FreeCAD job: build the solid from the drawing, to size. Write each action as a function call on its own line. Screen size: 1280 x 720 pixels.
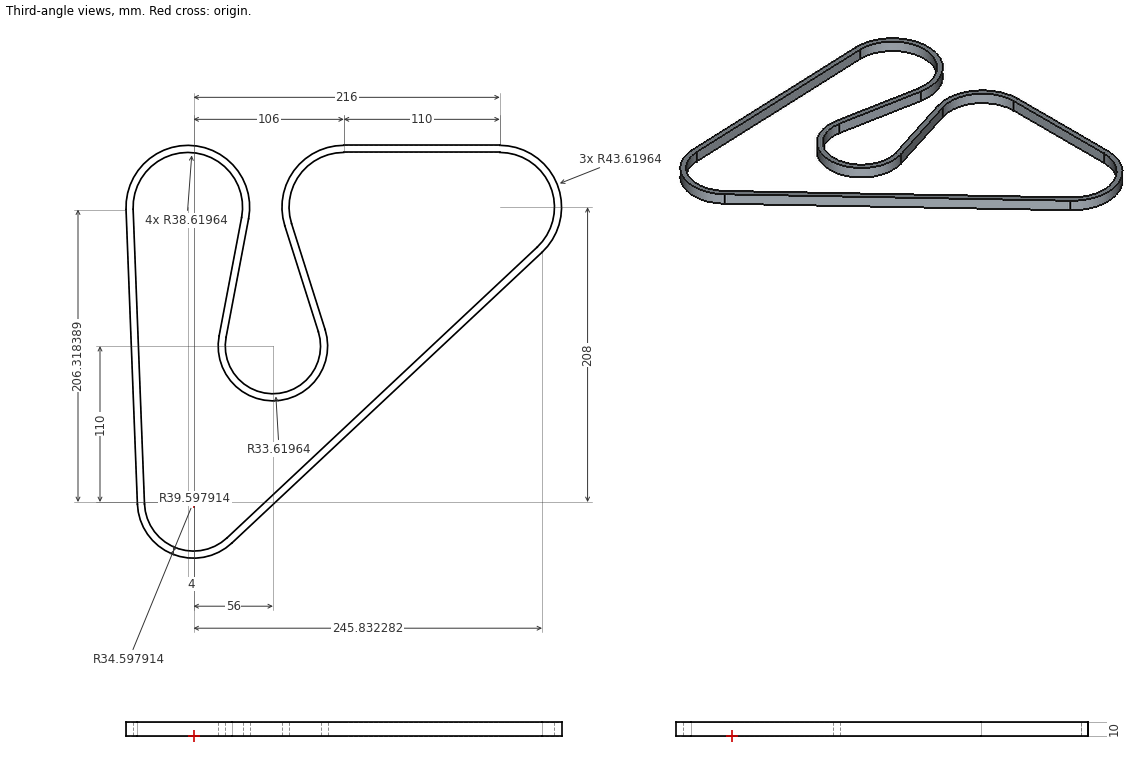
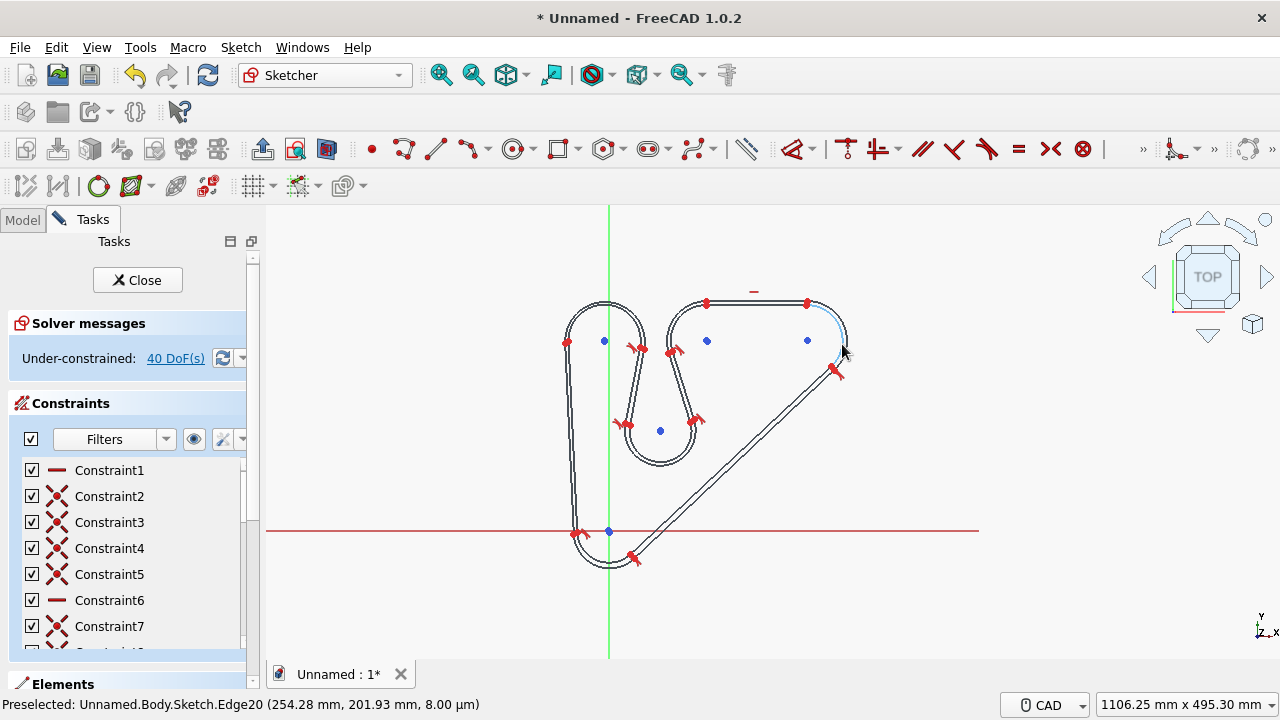
scroll(575, 475, up, 7)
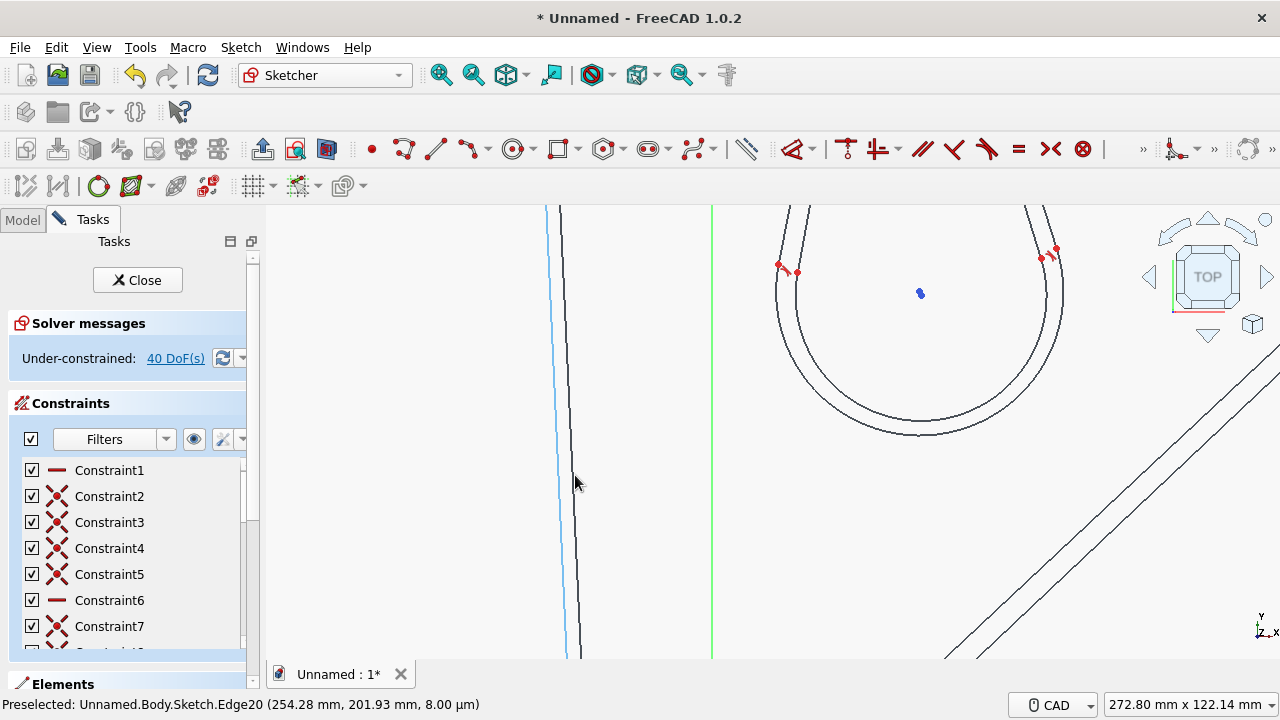
click(573, 473)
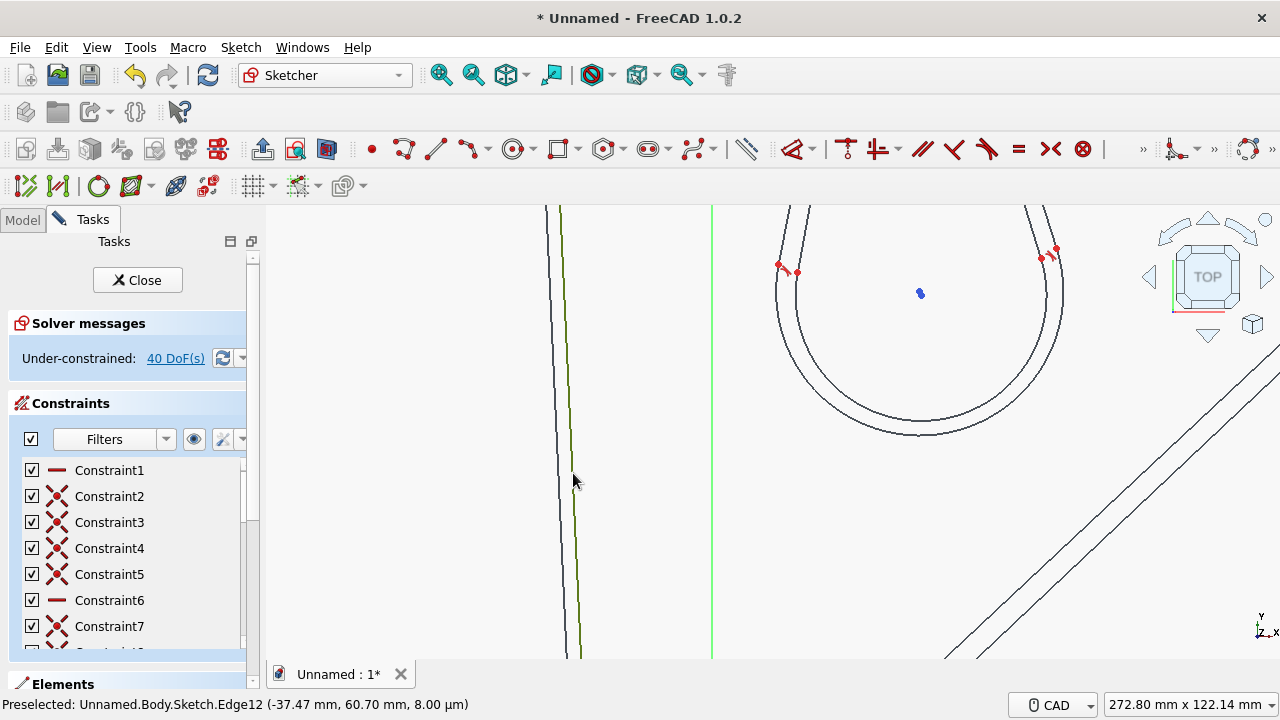
scroll(575, 475, down, 7)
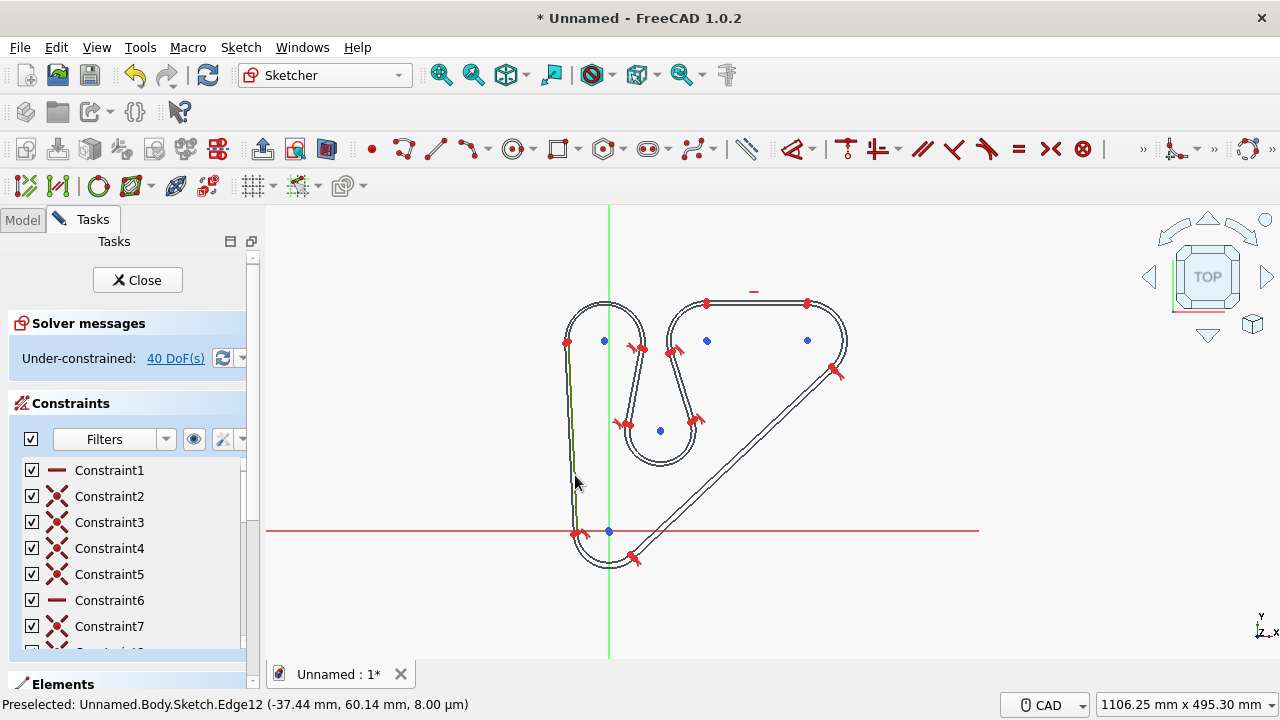
scroll(585, 552, up, 6)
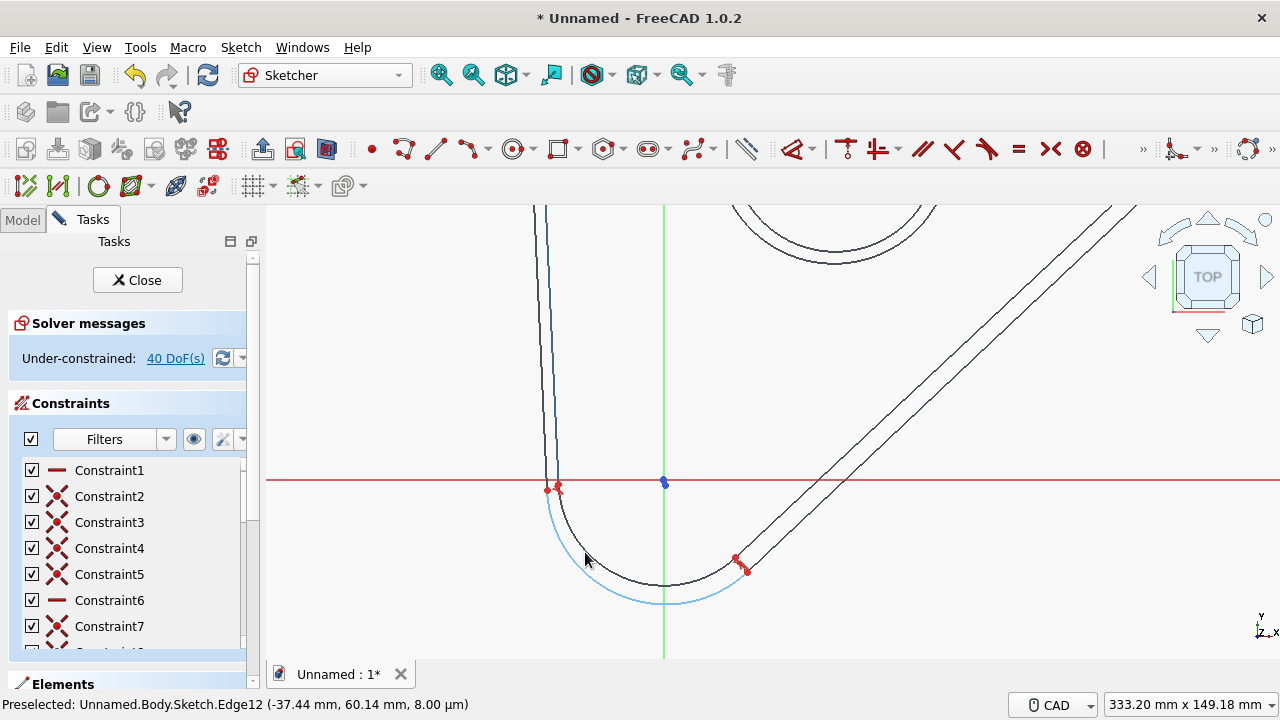
click(585, 550)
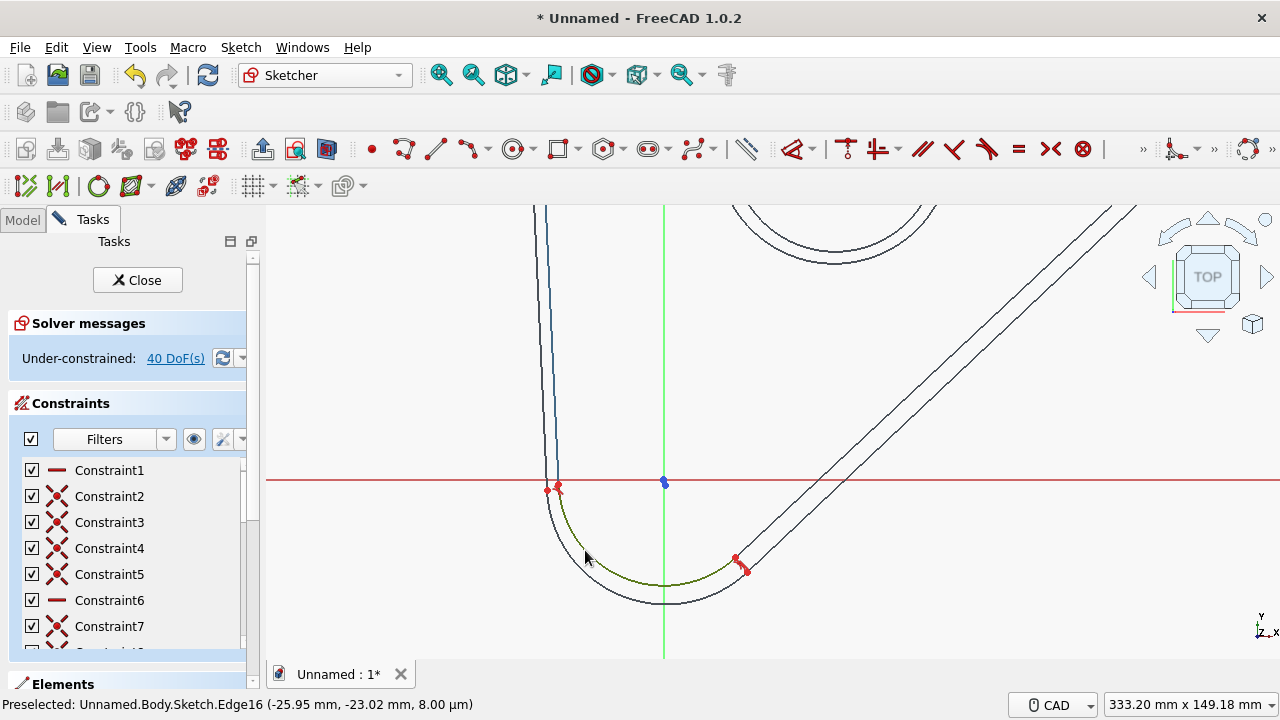
key(t)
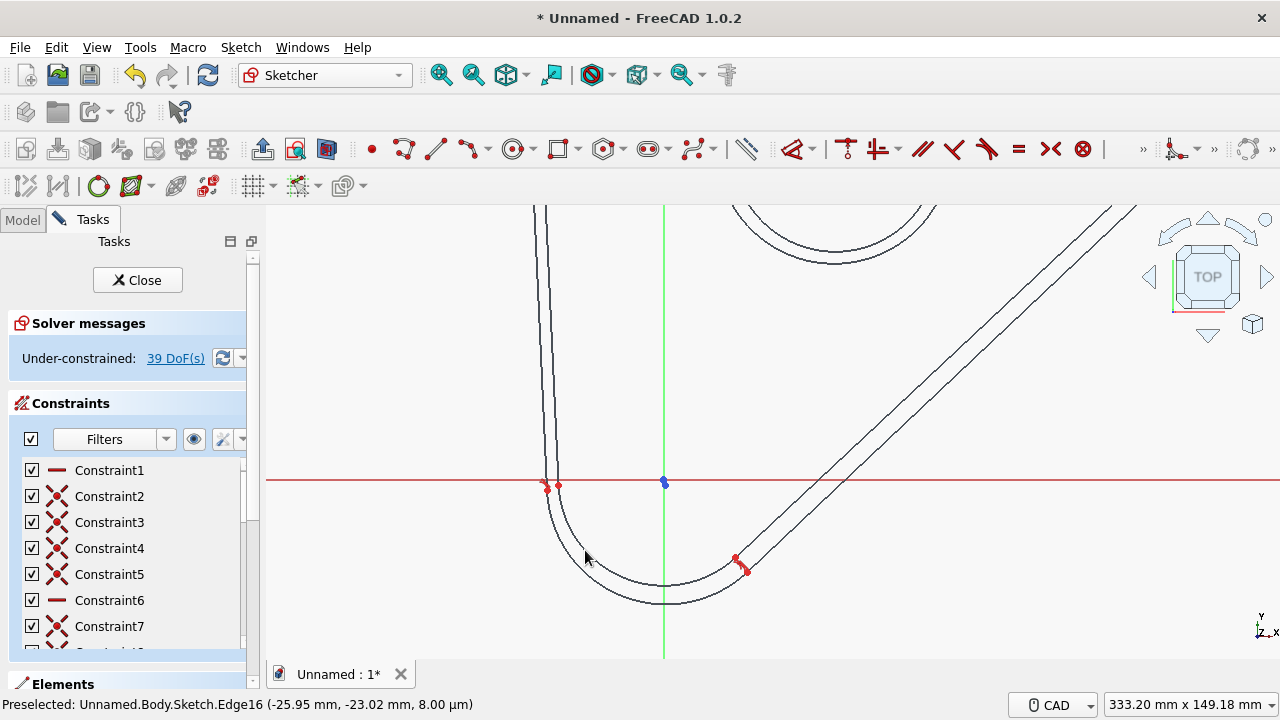
click(550, 295)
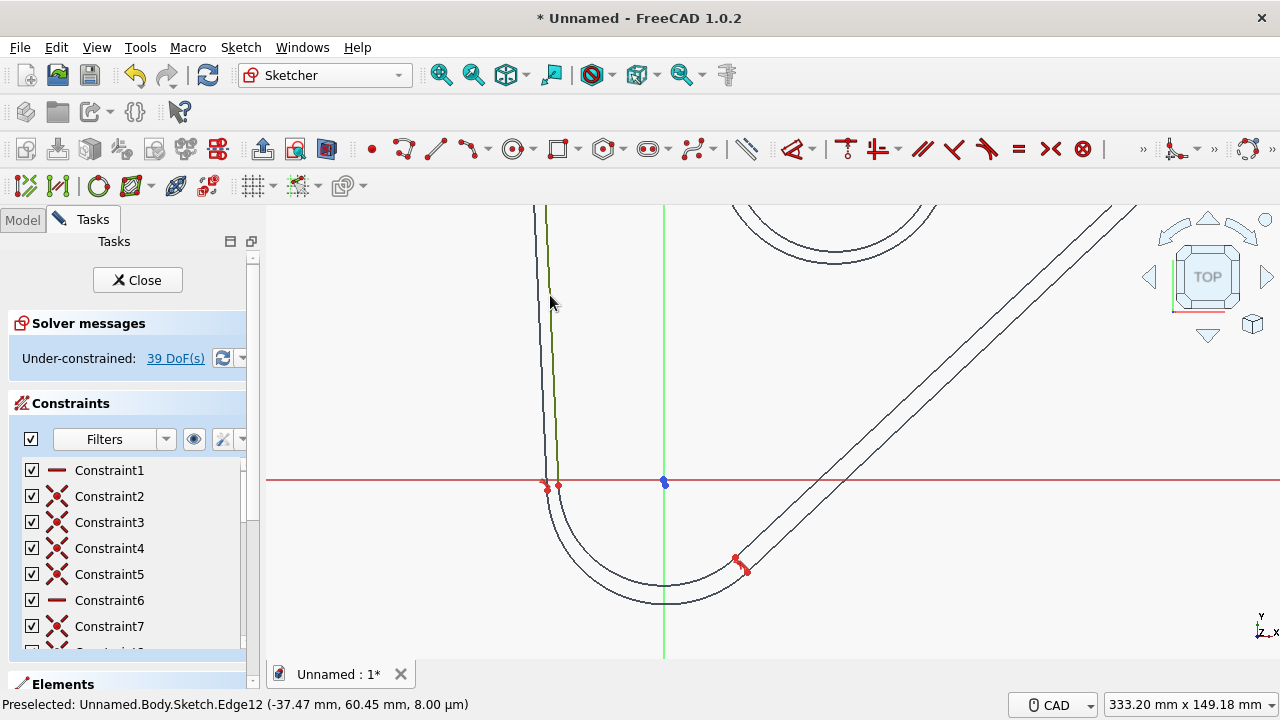
scroll(585, 552, down, 6)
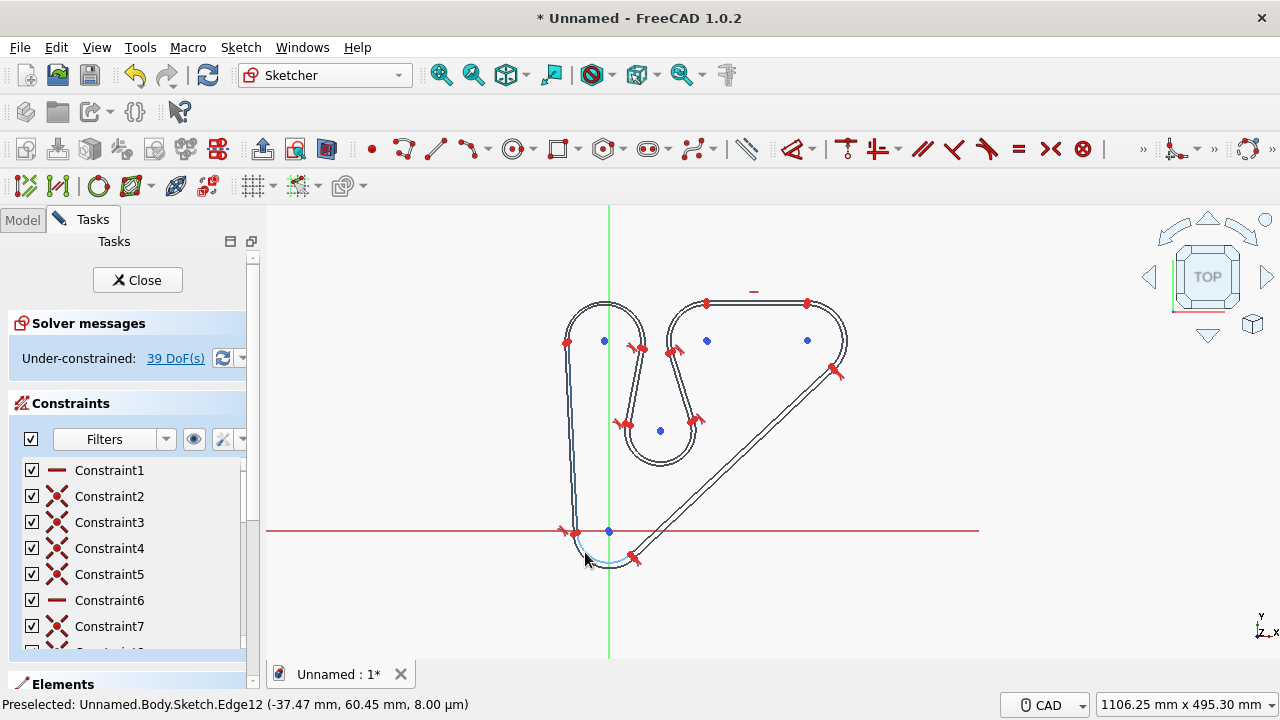
scroll(629, 314, up, 8)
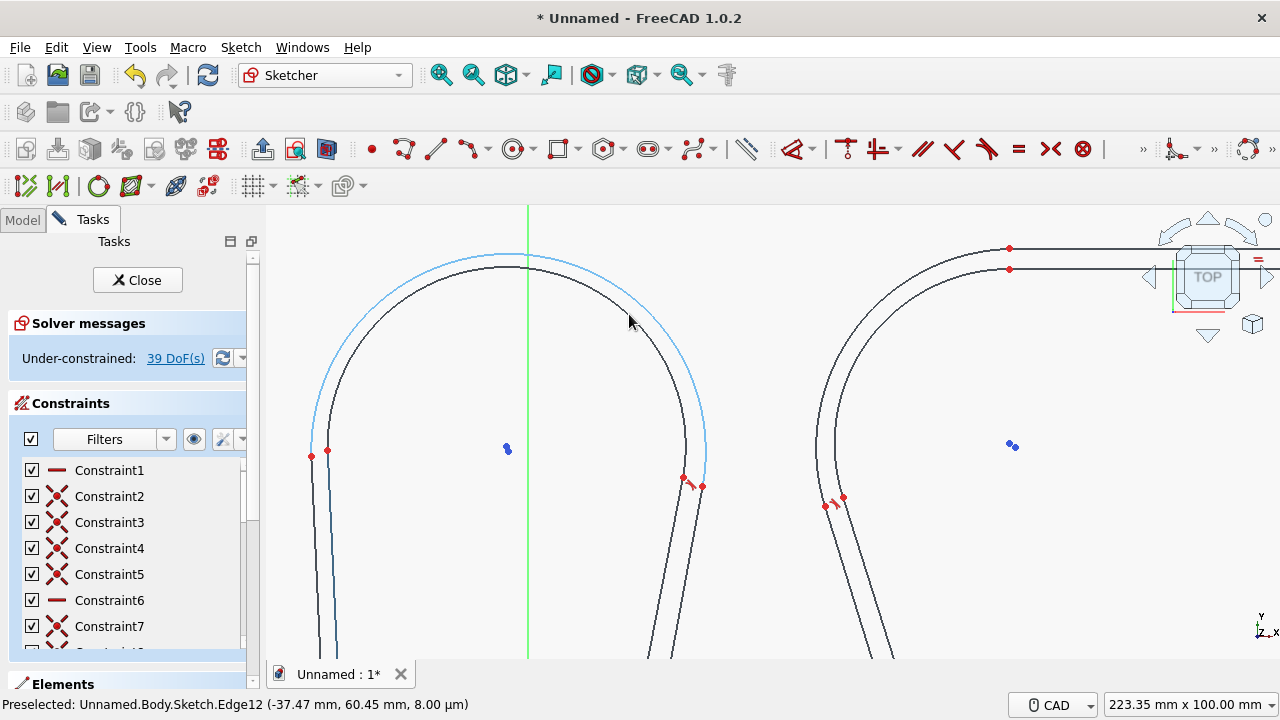
click(628, 314)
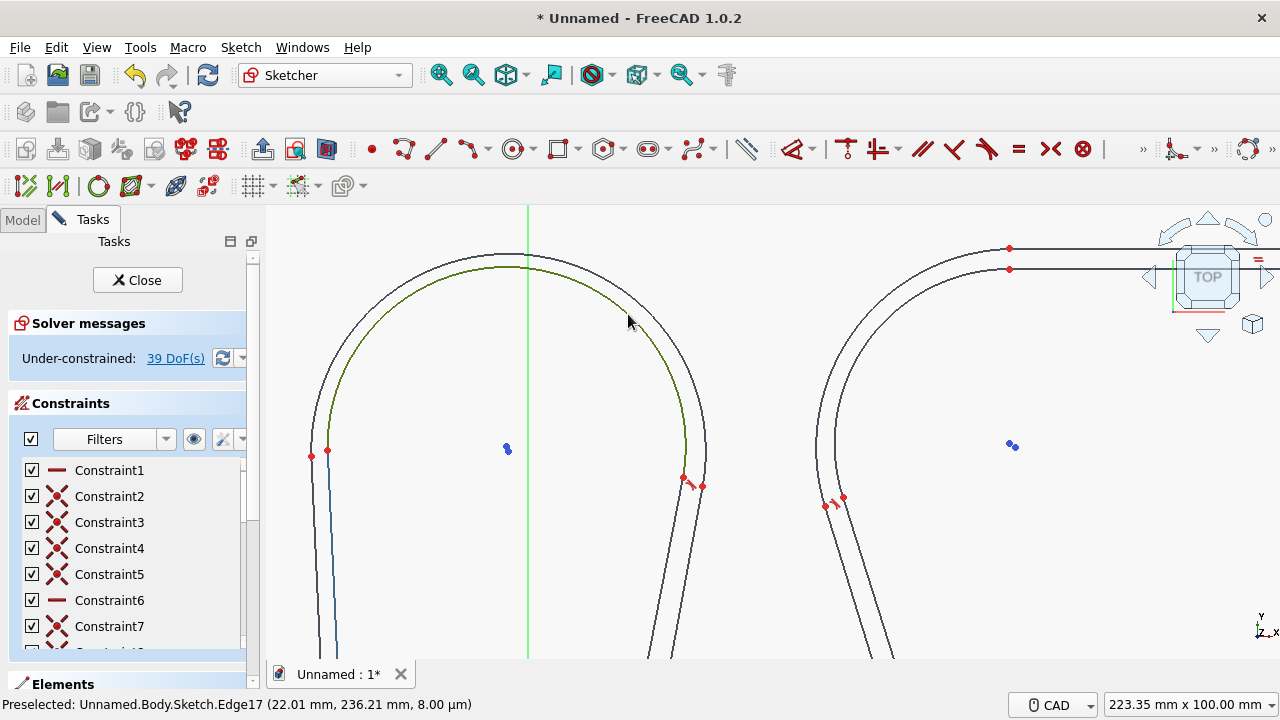
key(t)